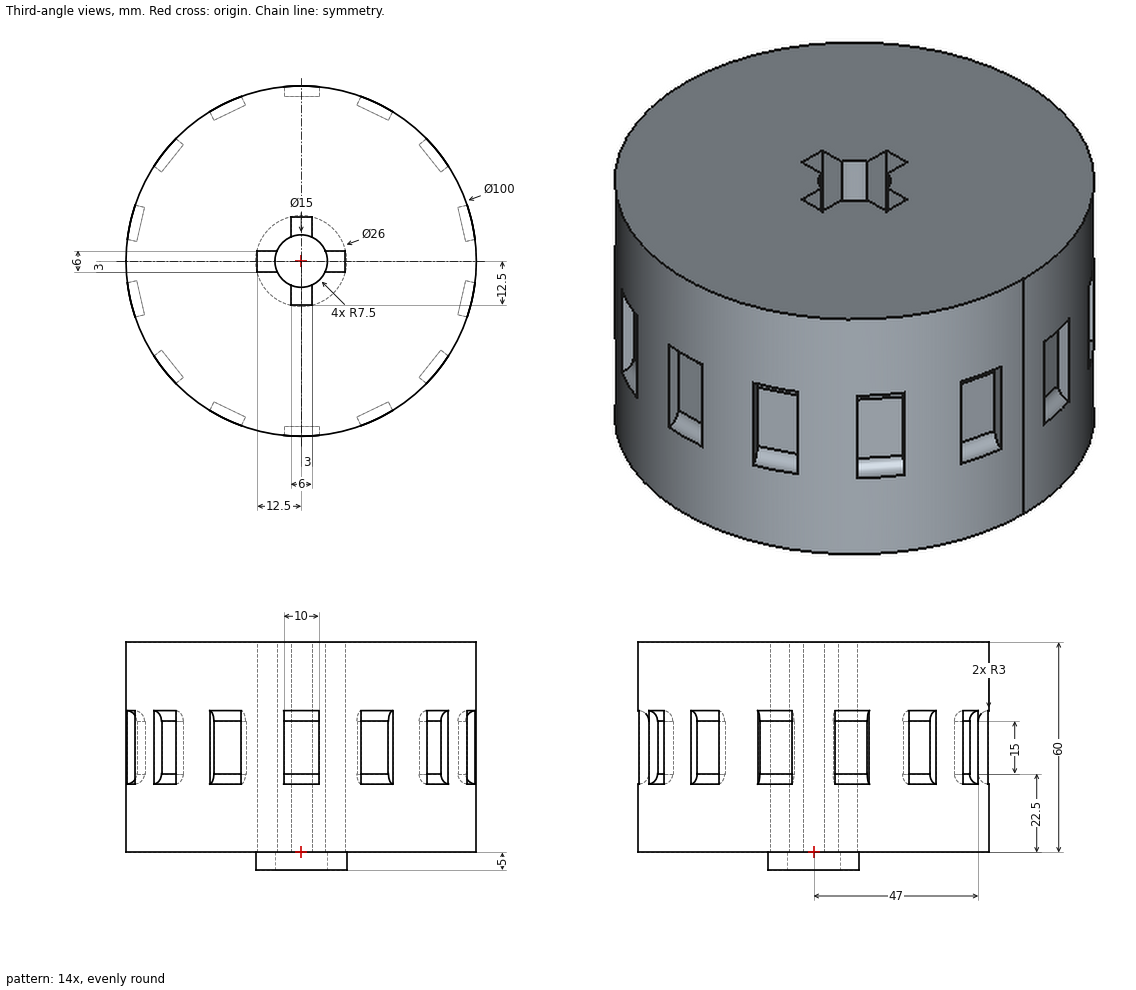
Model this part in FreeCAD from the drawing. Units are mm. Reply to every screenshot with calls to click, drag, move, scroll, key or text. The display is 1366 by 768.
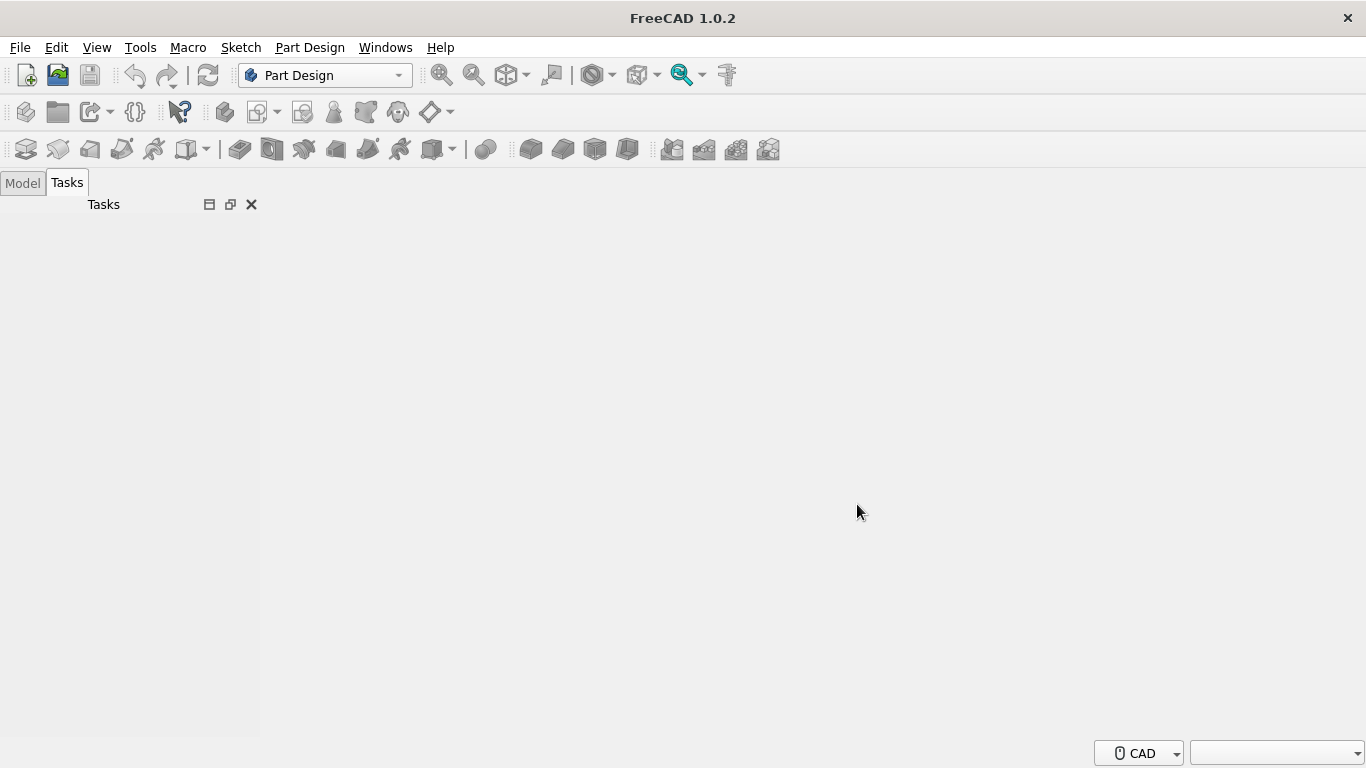
click(26, 76)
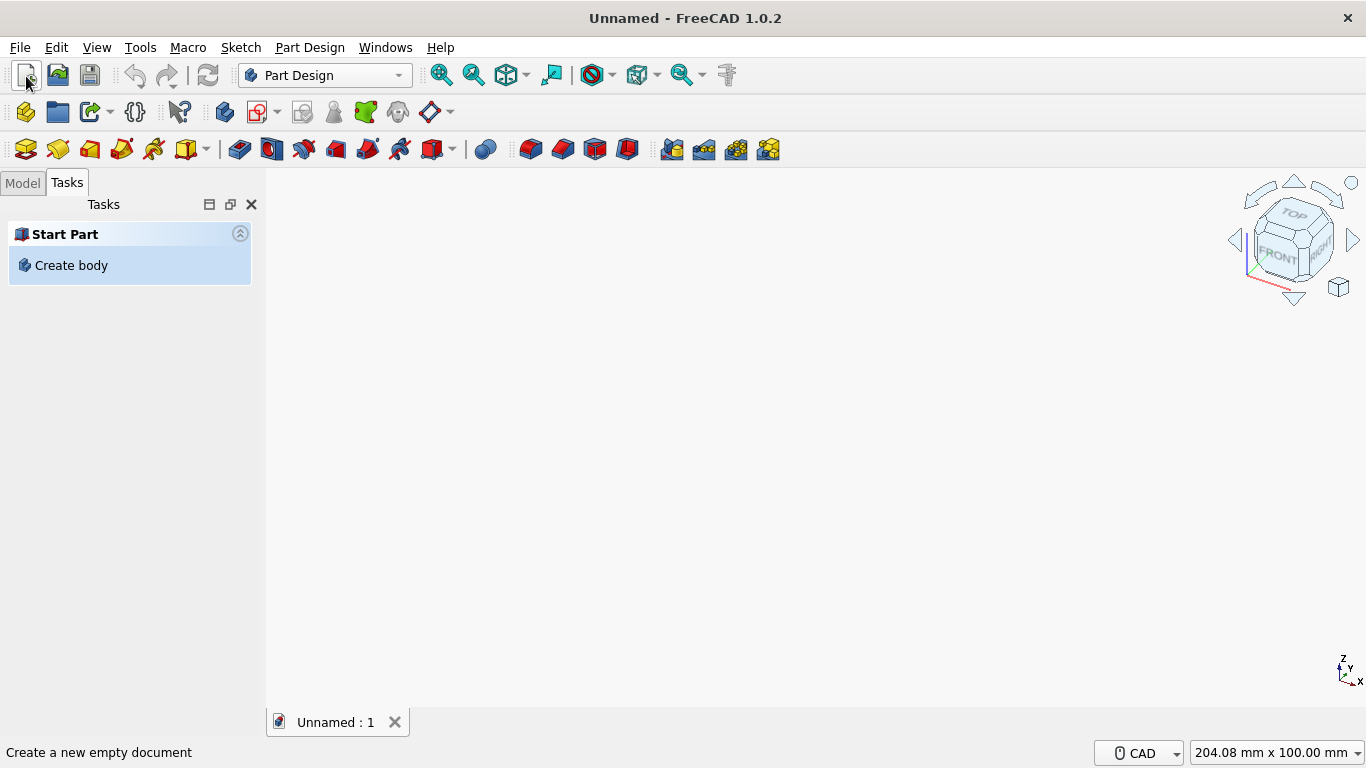
click(258, 112)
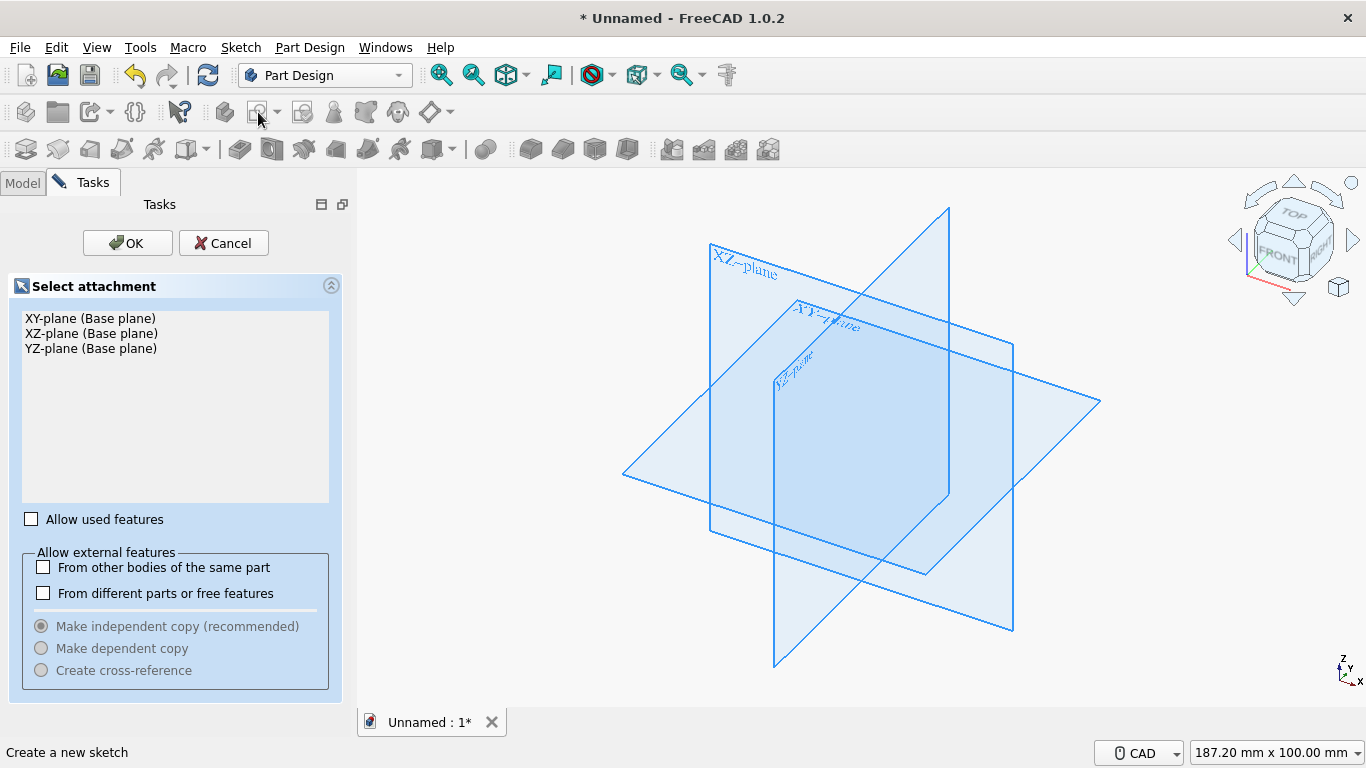
click(82, 318)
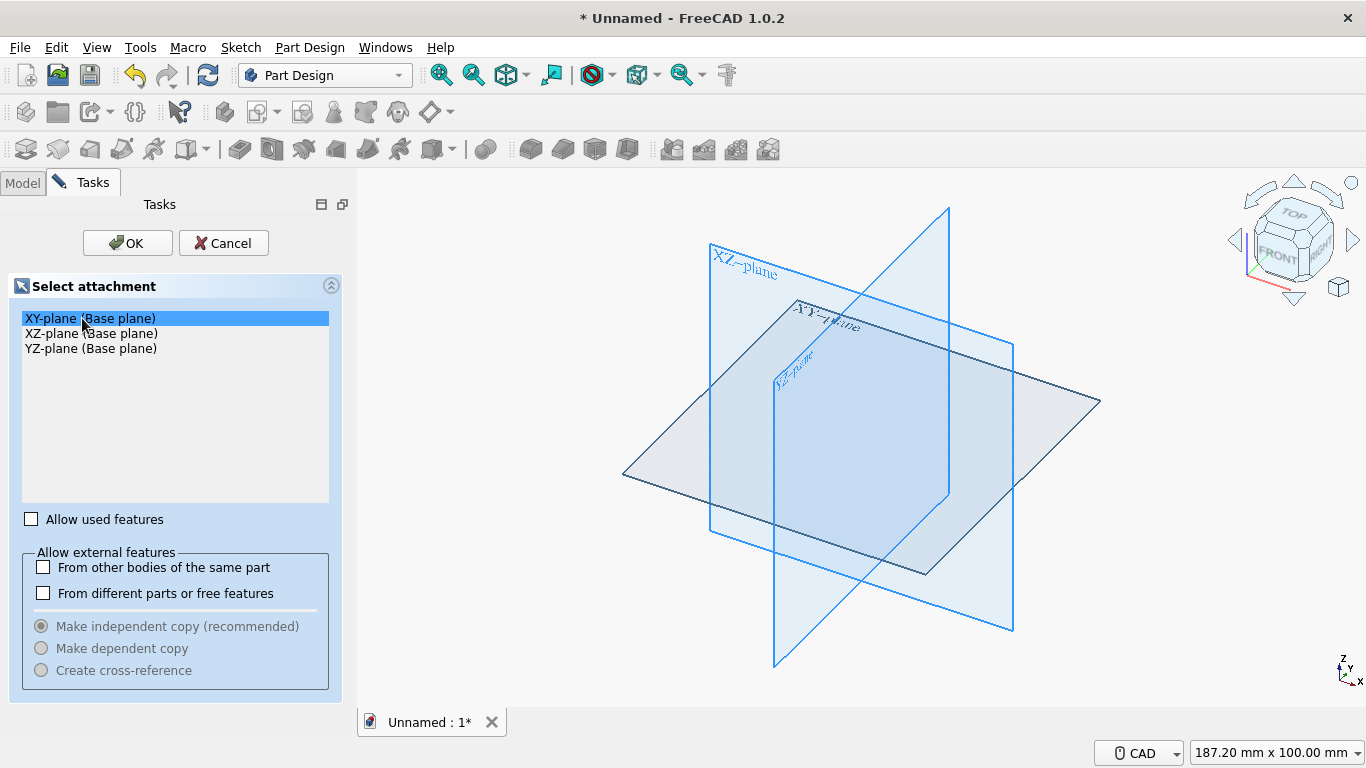
click(128, 243)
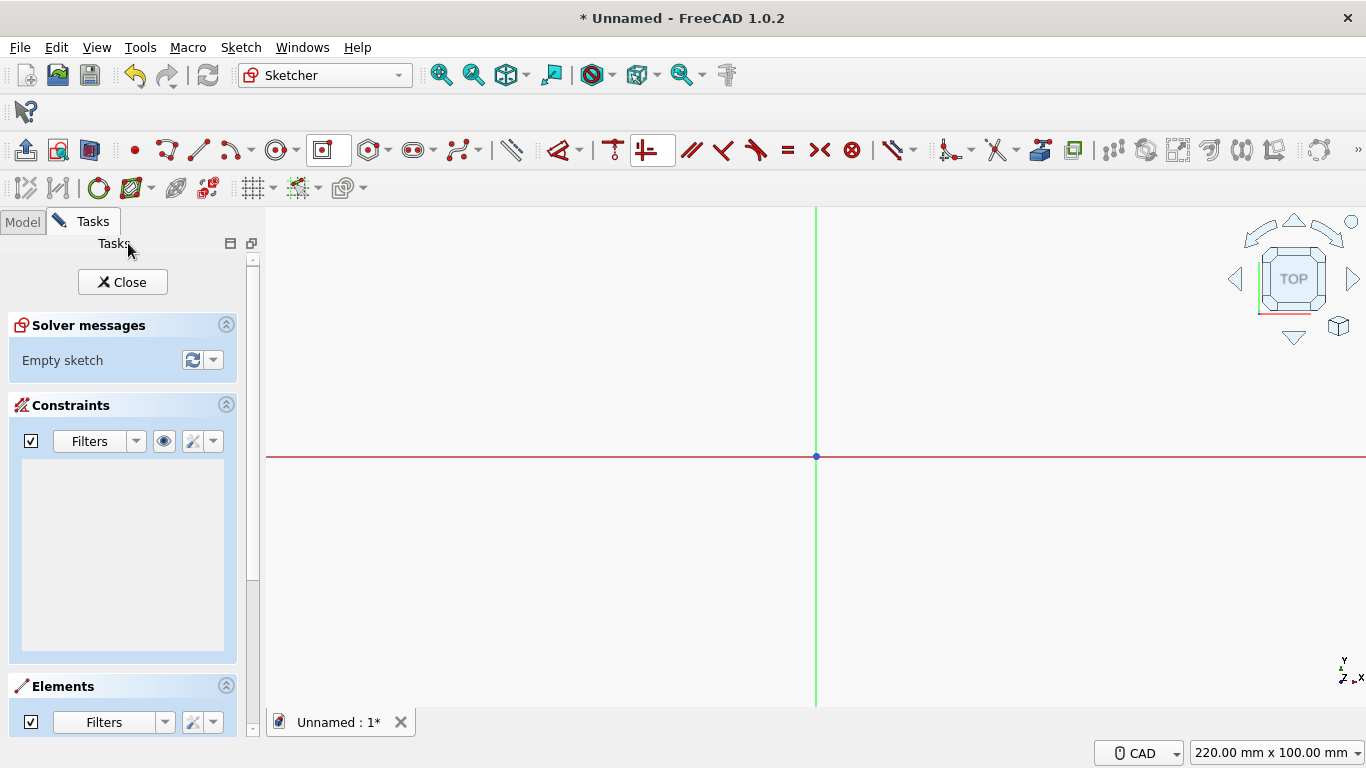
scroll(608, 457, down, 2)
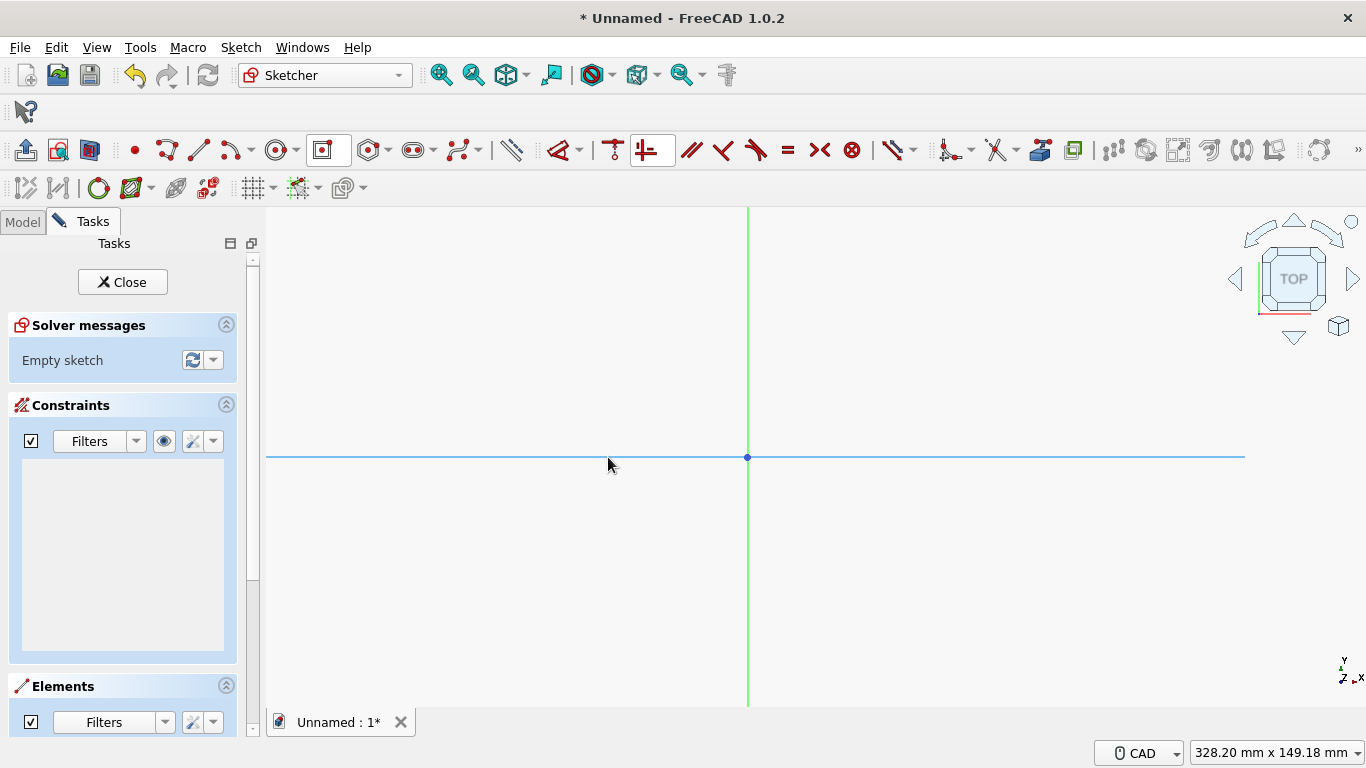
key(g)
key(m)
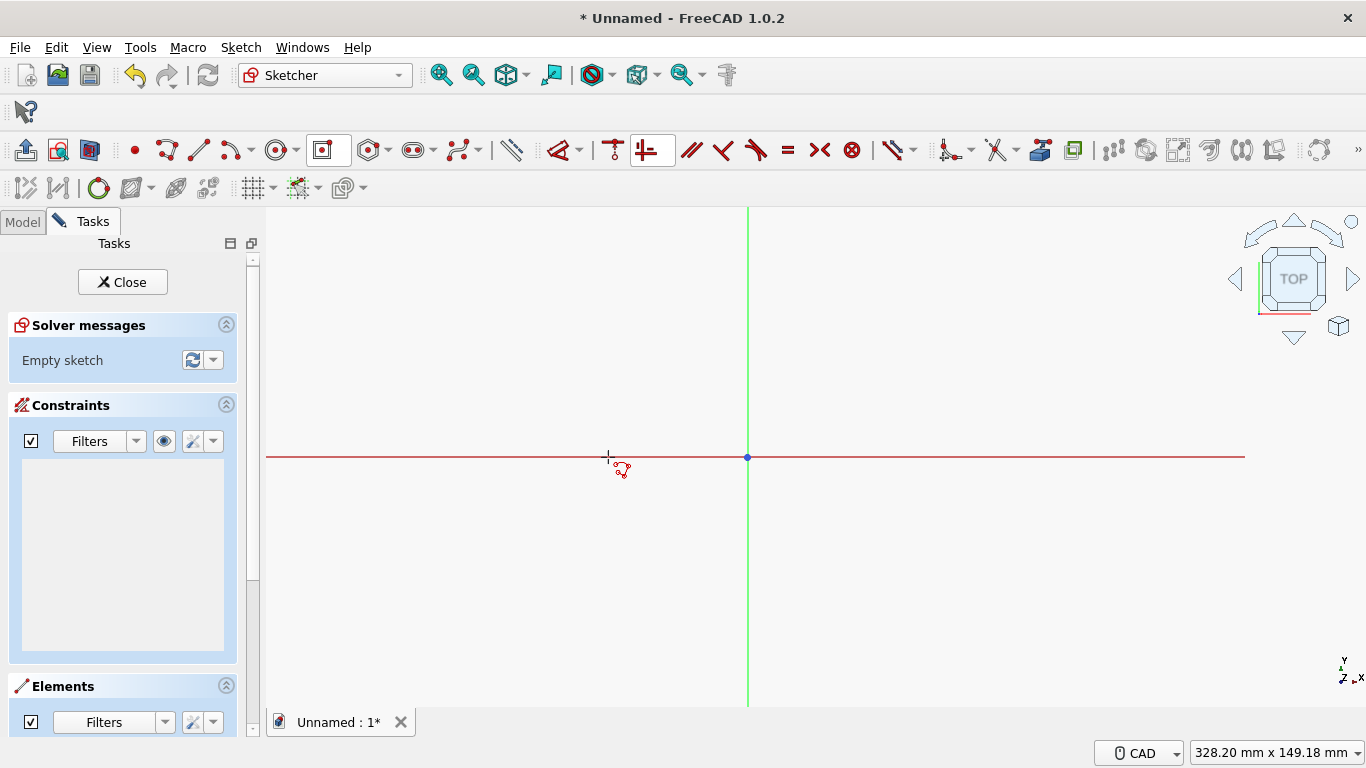
scroll(758, 480, up, 3)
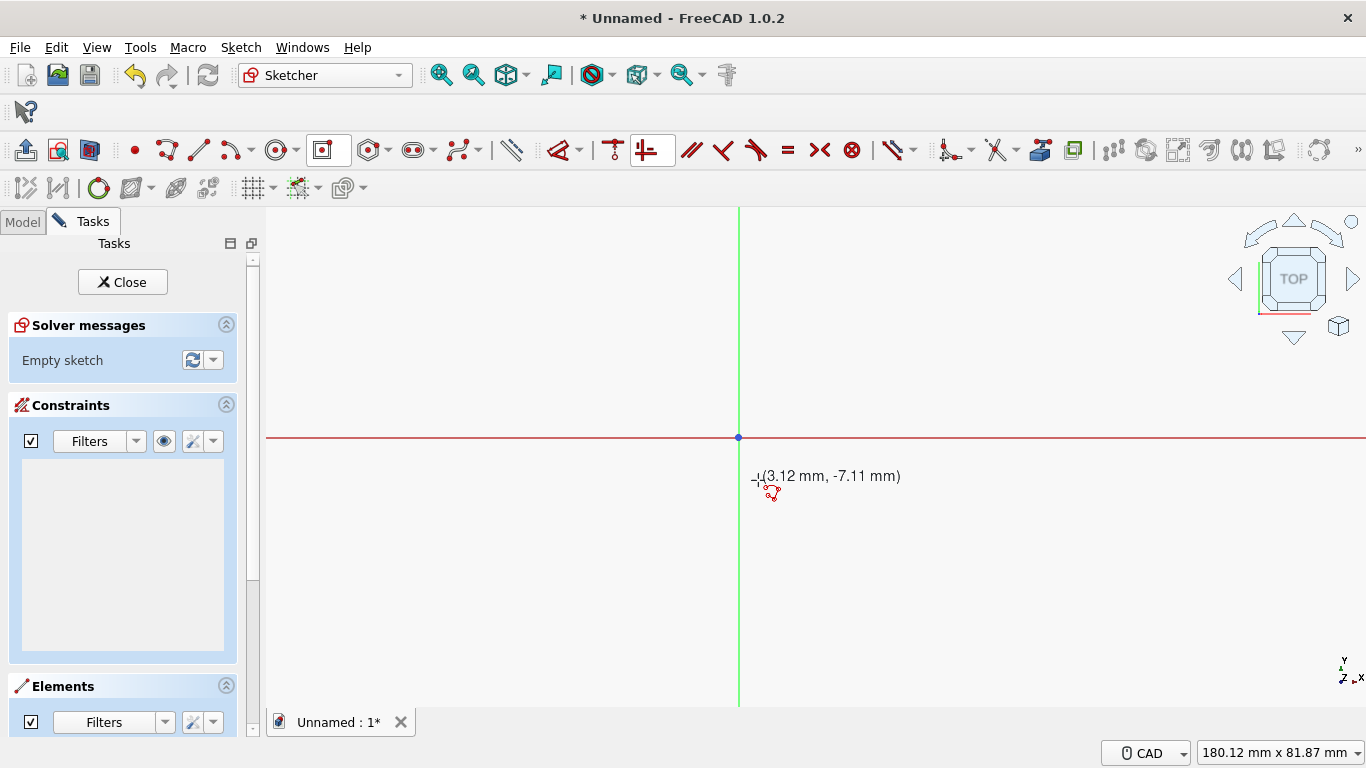
click(757, 480)
click(757, 514)
click(720, 514)
click(720, 480)
right_click(720, 480)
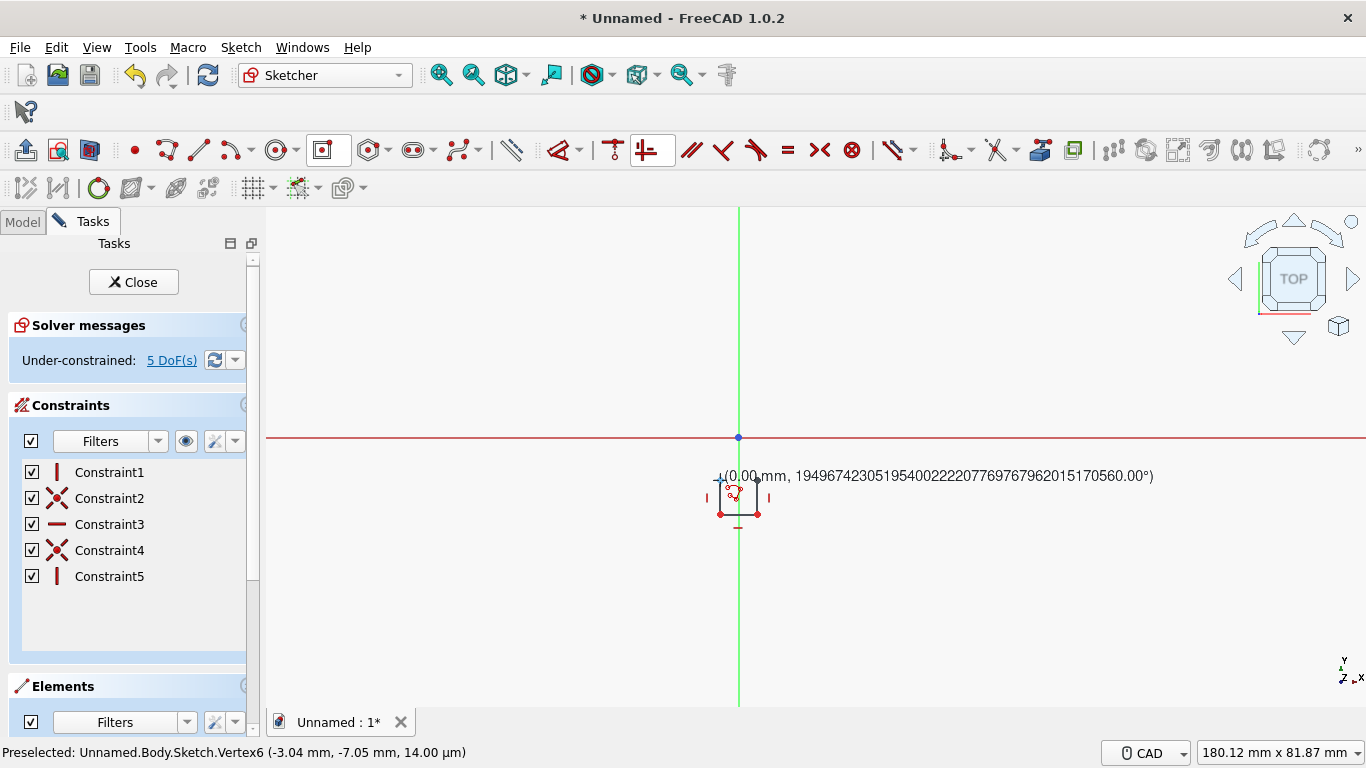
click(697, 456)
click(662, 456)
click(662, 420)
click(697, 420)
right_click(697, 420)